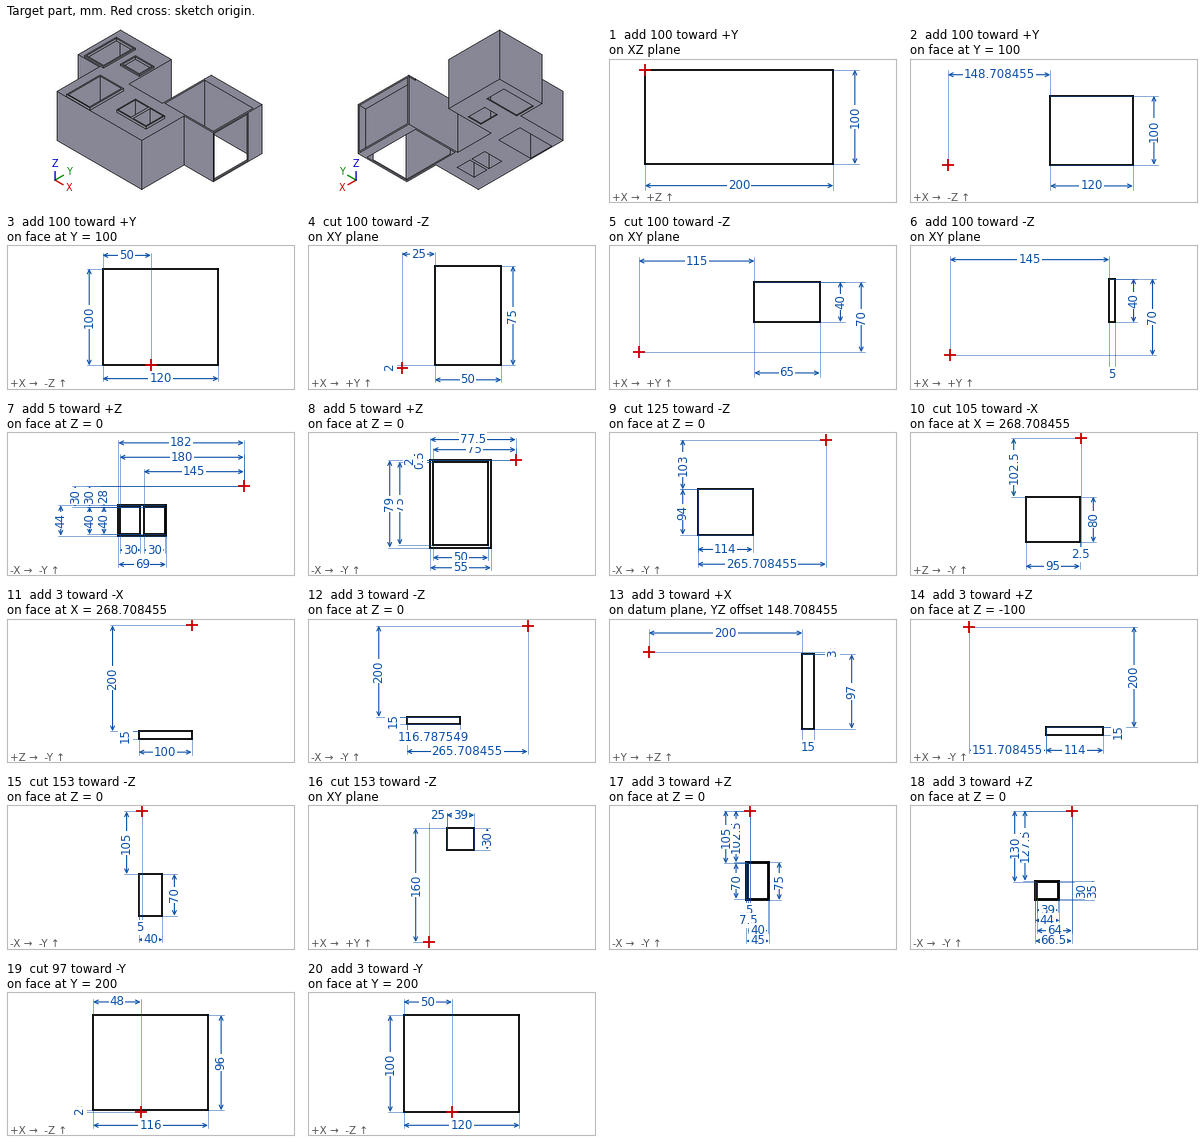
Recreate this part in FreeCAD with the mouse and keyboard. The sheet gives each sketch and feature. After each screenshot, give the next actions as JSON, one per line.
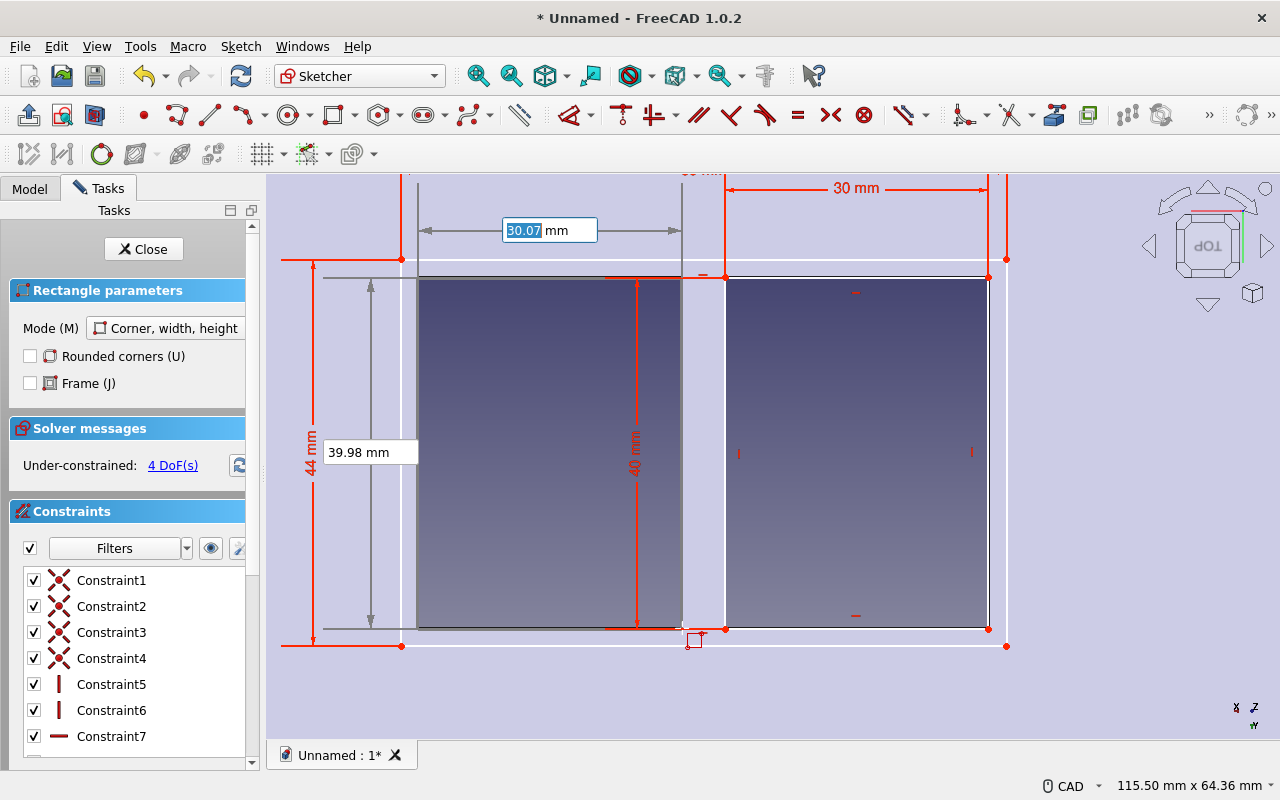
{"action": "type", "text": "30"}
{"action": "key", "text": "Tab"}
{"action": "type", "text": "40"}
{"action": "key", "text": "Return"}
{"action": "key", "text": "Escape"}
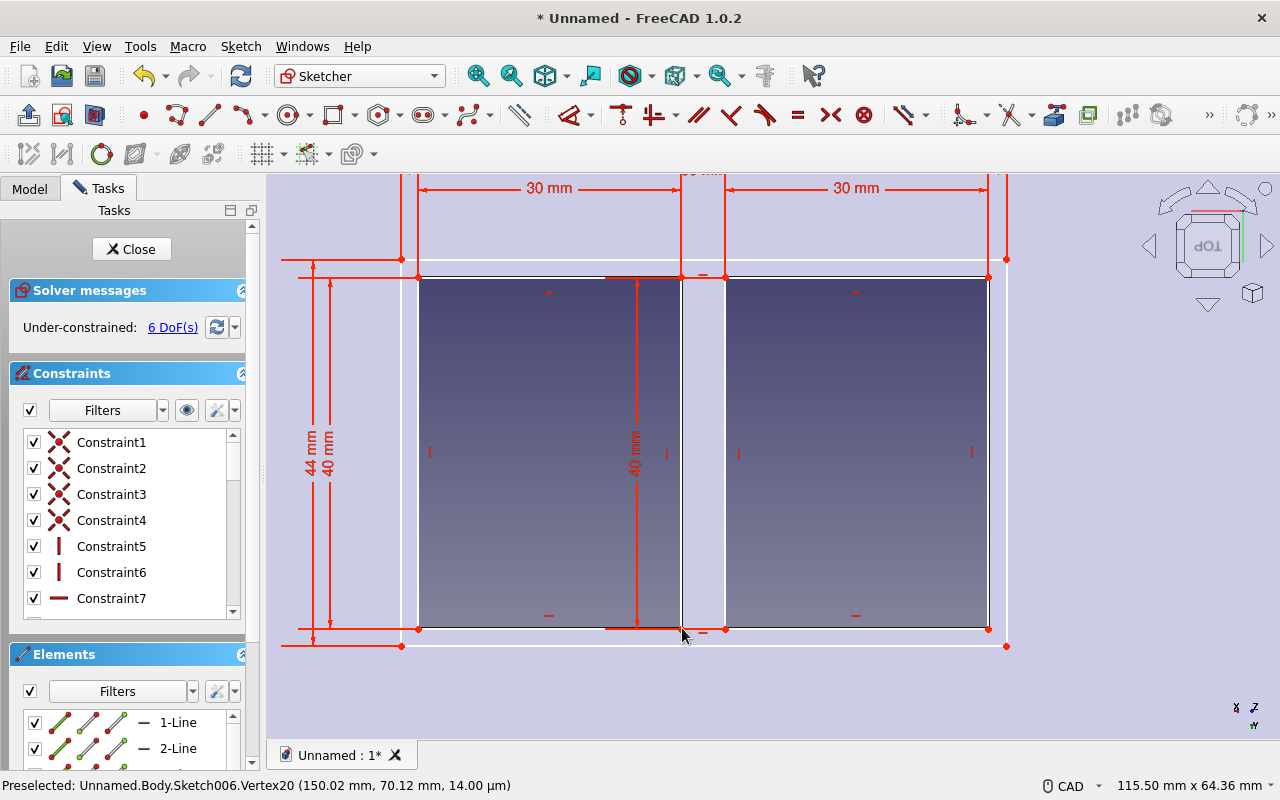
{"action": "left_click", "coordinate": [568, 116]}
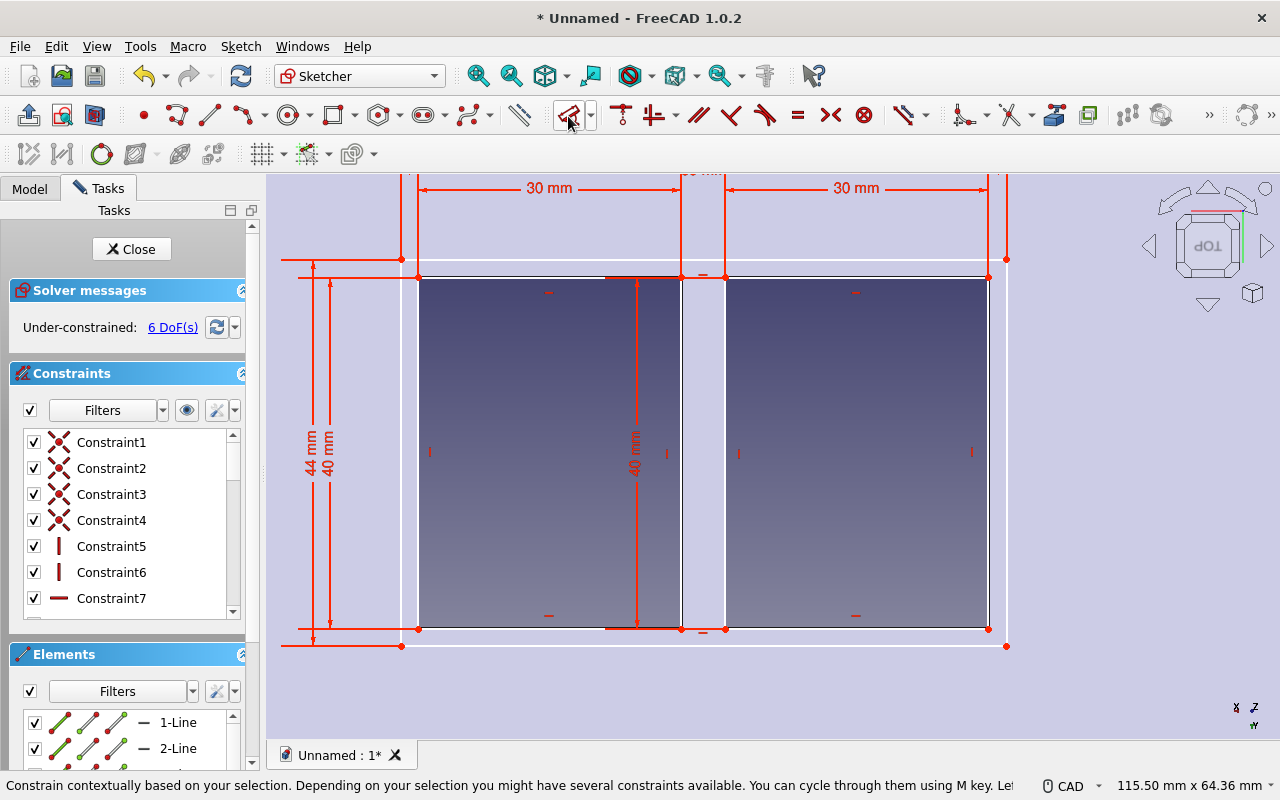
{"action": "left_click", "coordinate": [401, 260]}
{"action": "left_click", "coordinate": [367, 231]}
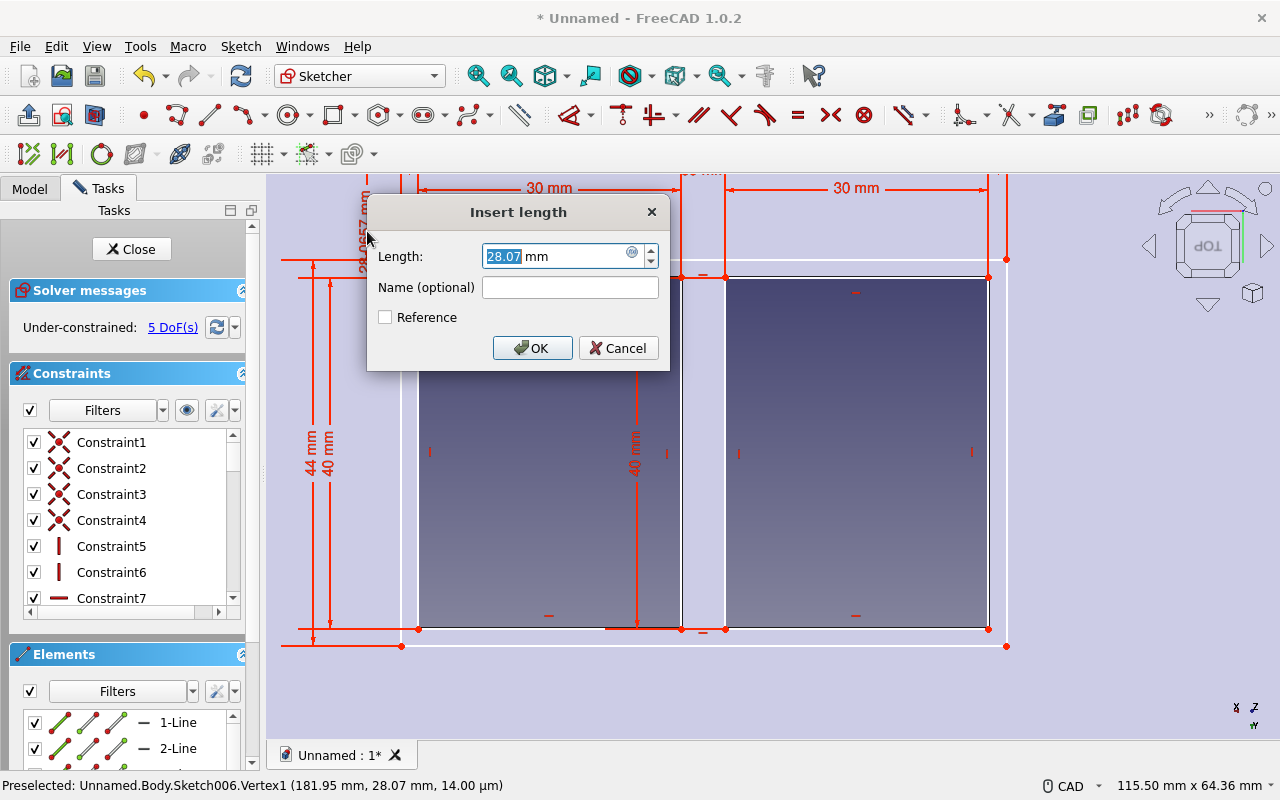
{"action": "type", "text": "28"}
{"action": "key", "text": "Return"}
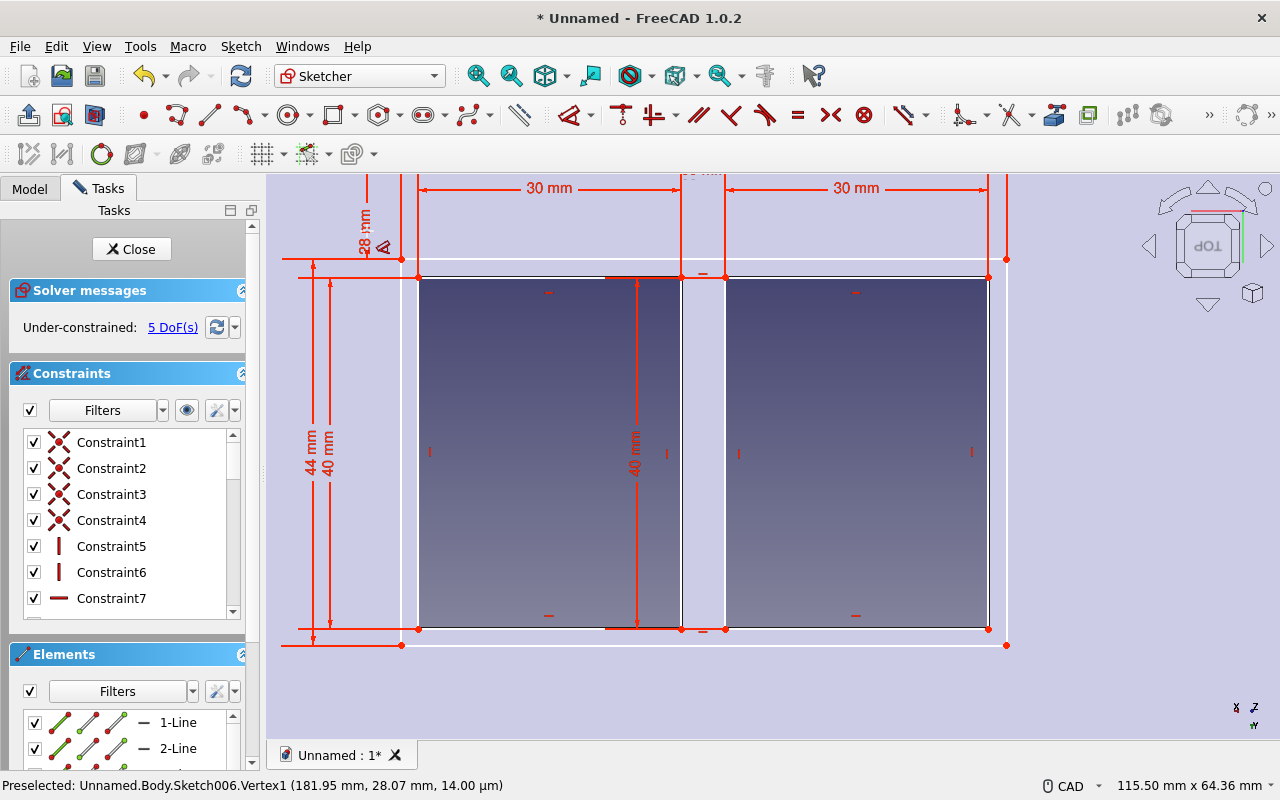
{"action": "left_click", "coordinate": [725, 278]}
{"action": "left_click", "coordinate": [691, 240]}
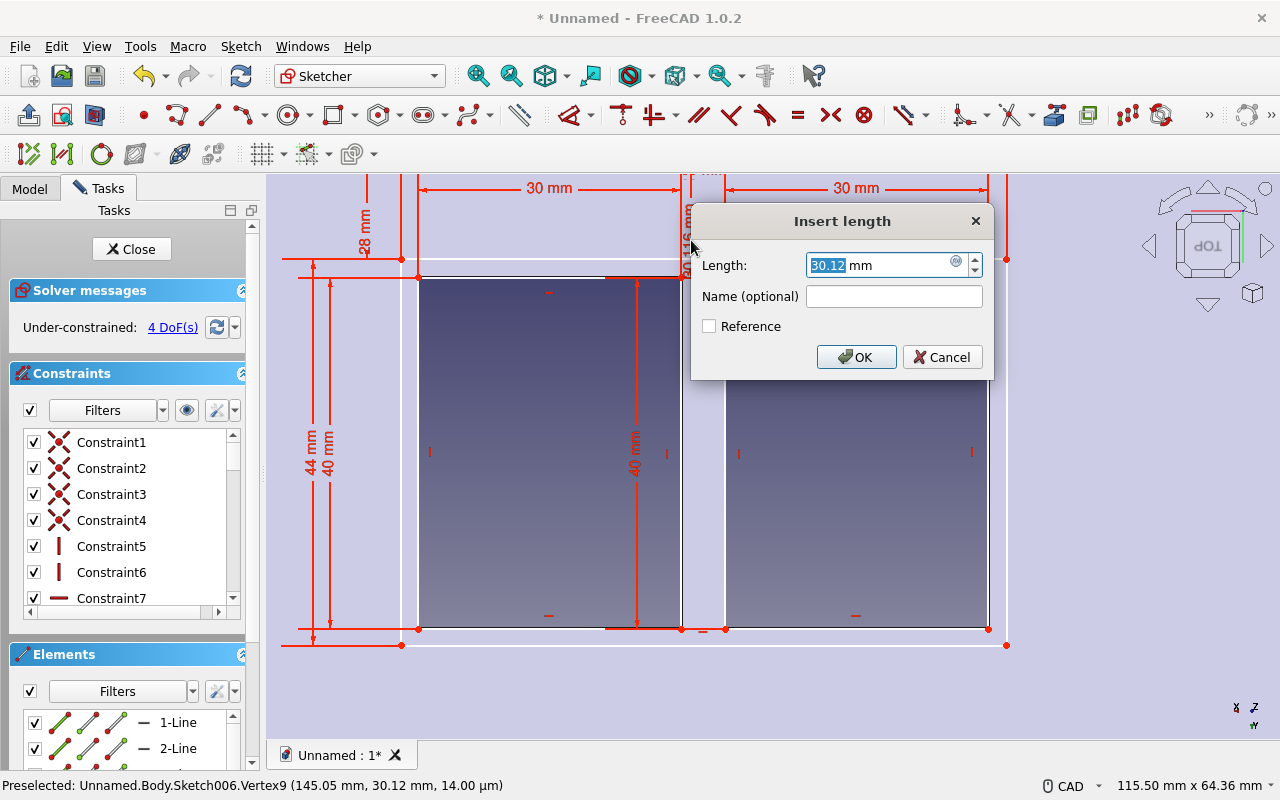
{"action": "type", "text": "30"}
{"action": "key", "text": "Return"}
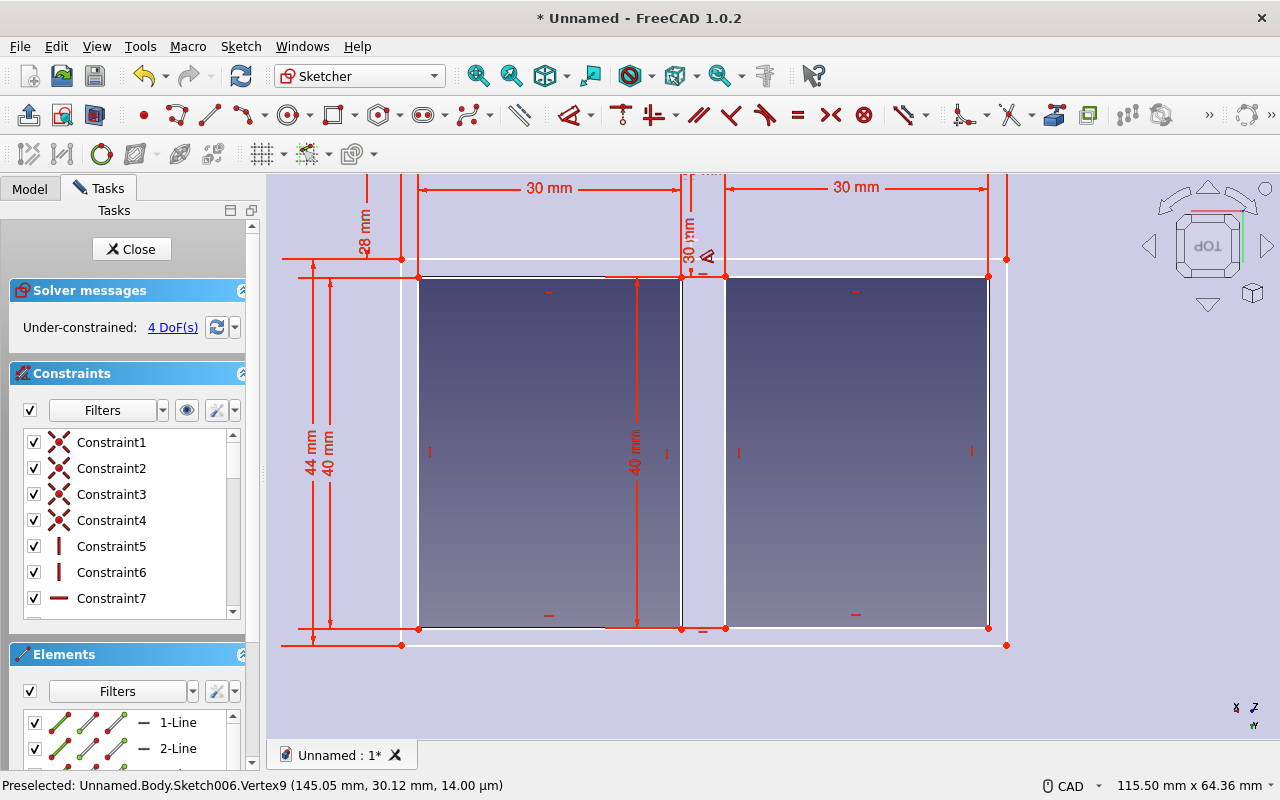
{"action": "left_click", "coordinate": [418, 278]}
{"action": "left_click", "coordinate": [384, 257]}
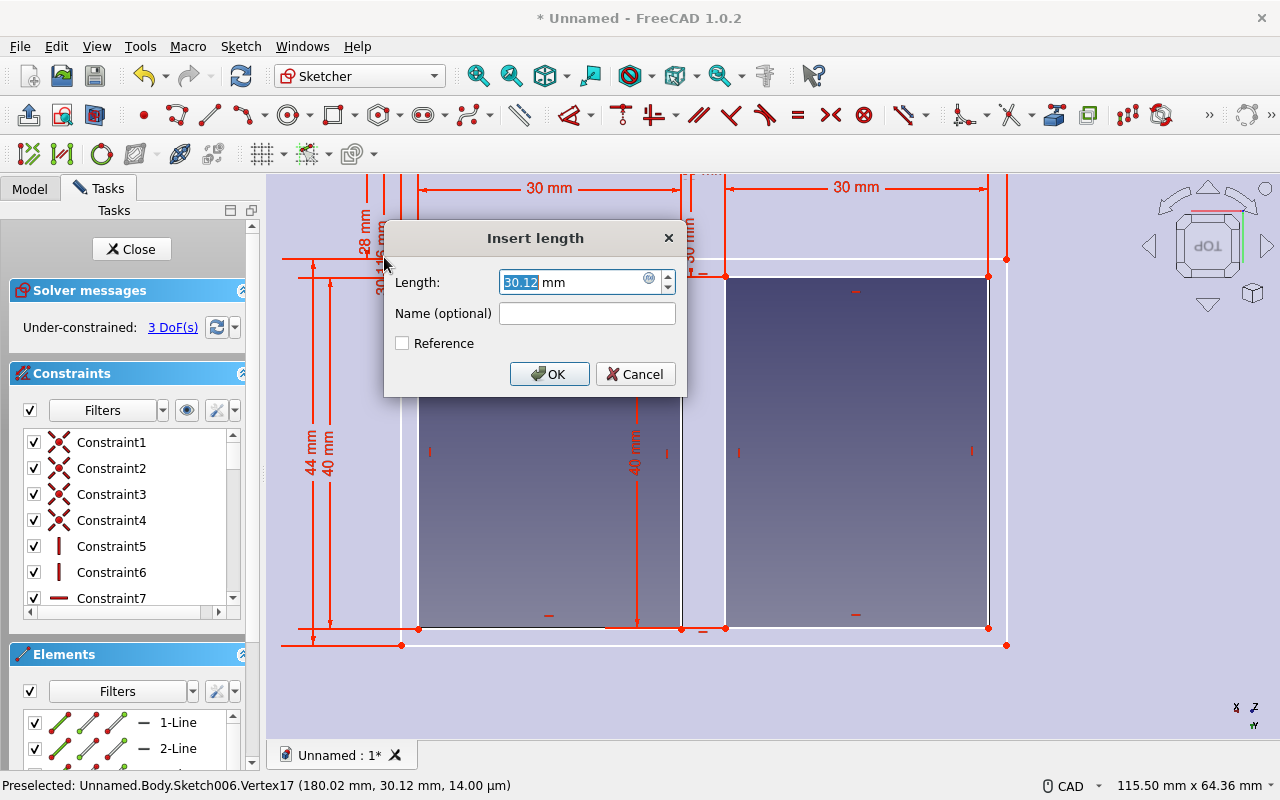
{"action": "type", "text": "30"}
{"action": "key", "text": "Return"}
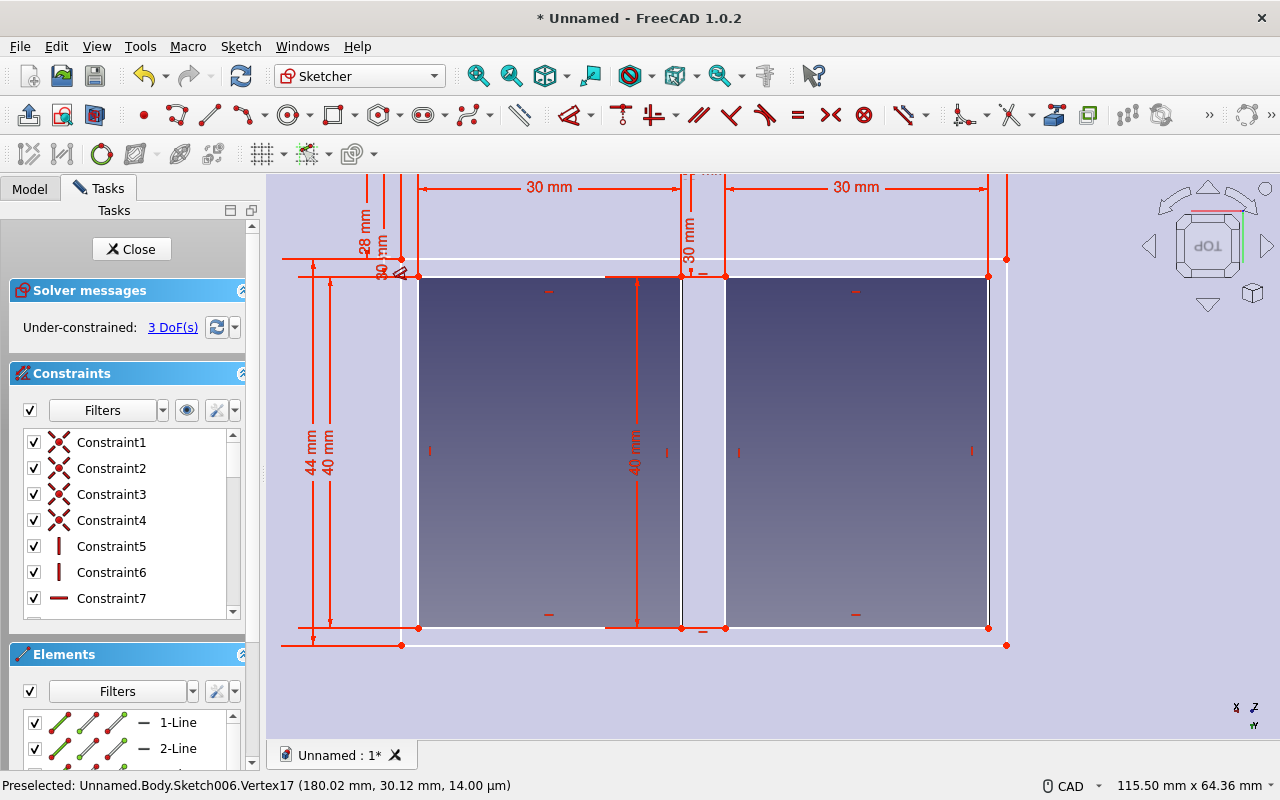
{"action": "left_click", "coordinate": [401, 259]}
{"action": "left_click", "coordinate": [758, 293]}